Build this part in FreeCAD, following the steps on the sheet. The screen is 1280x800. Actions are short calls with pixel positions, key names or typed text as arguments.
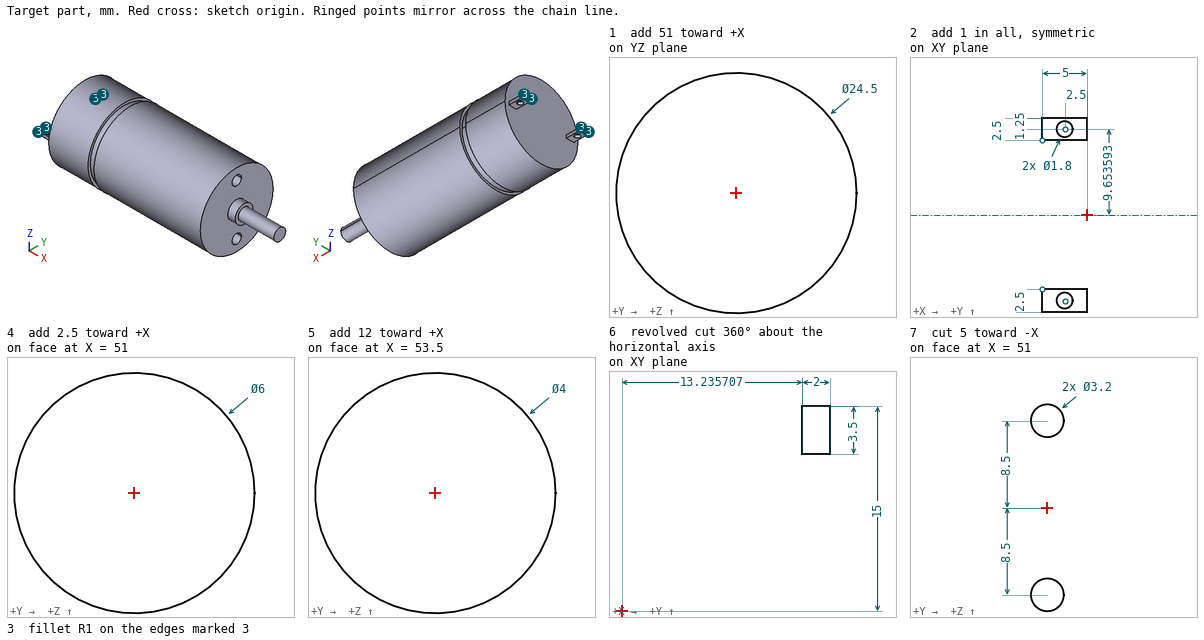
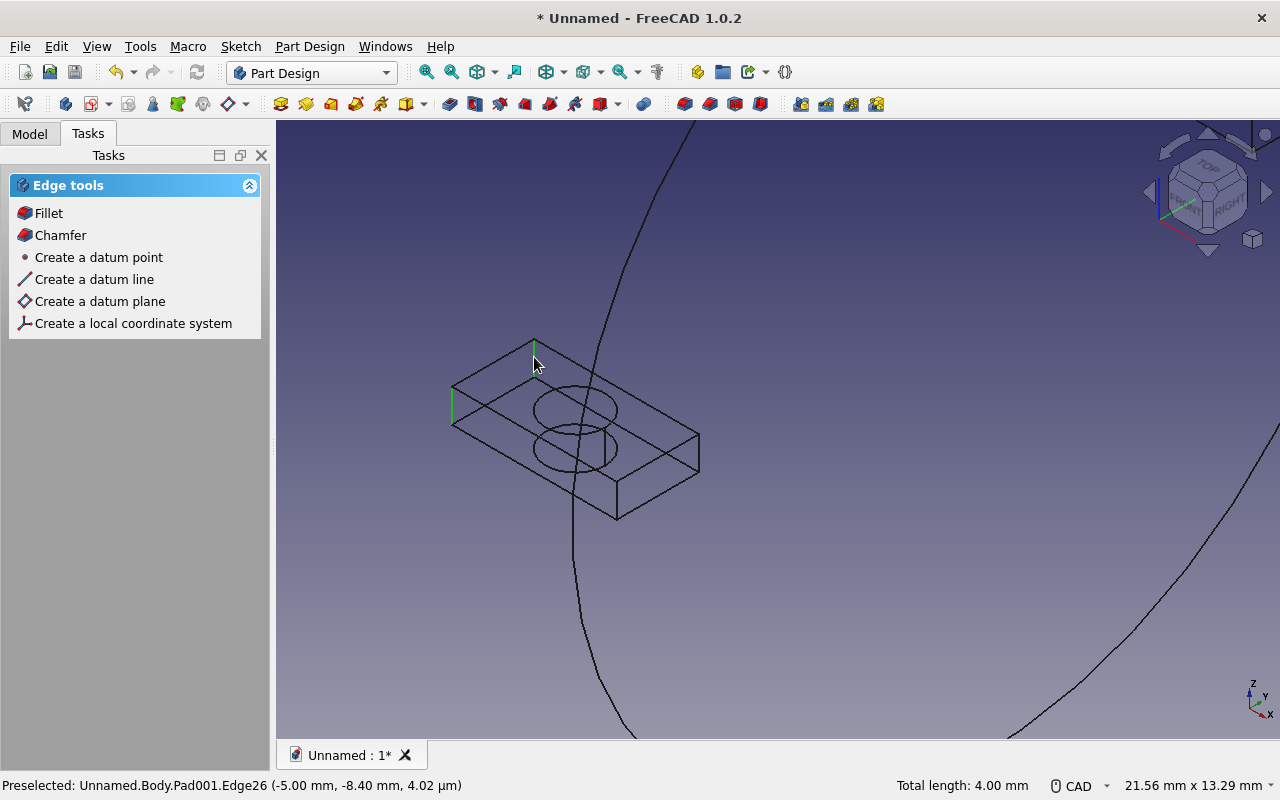
key(v)
key(1)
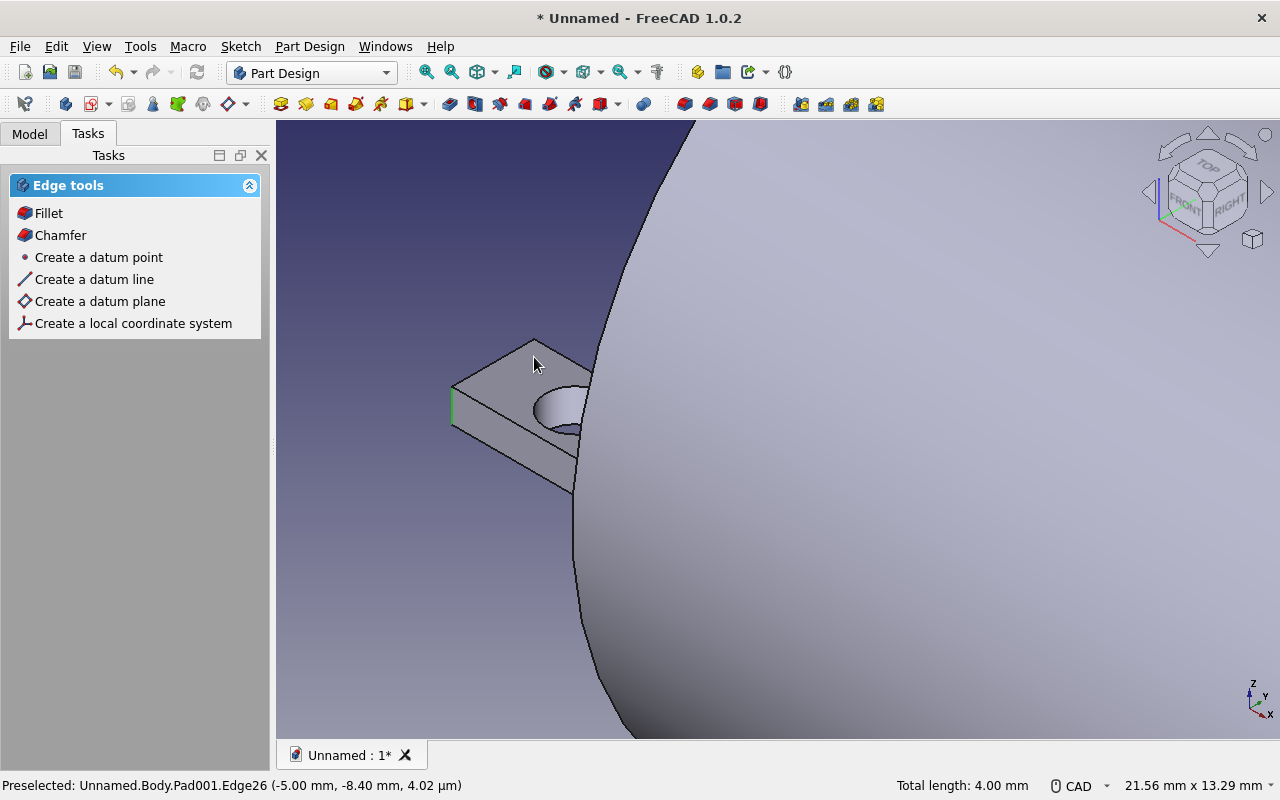
click(685, 104)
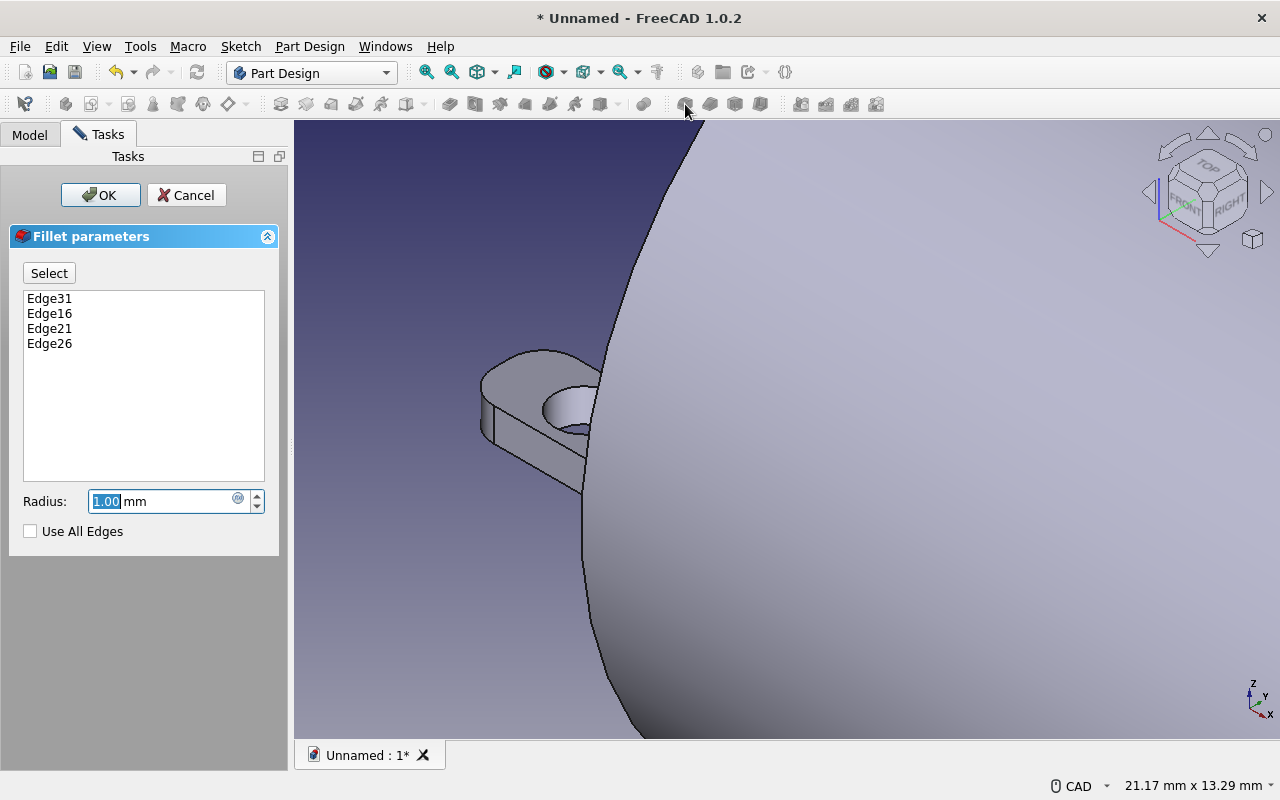
text(1)
key(Tab)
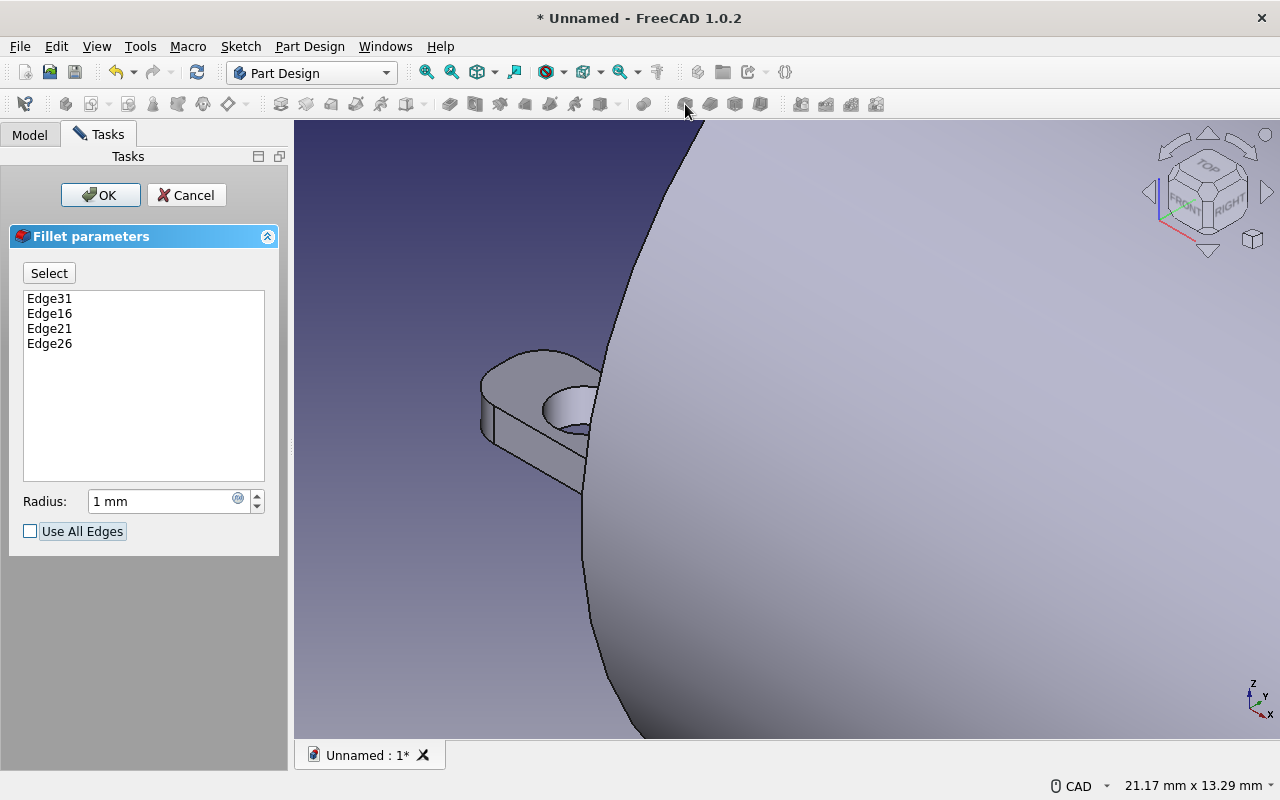
click(101, 195)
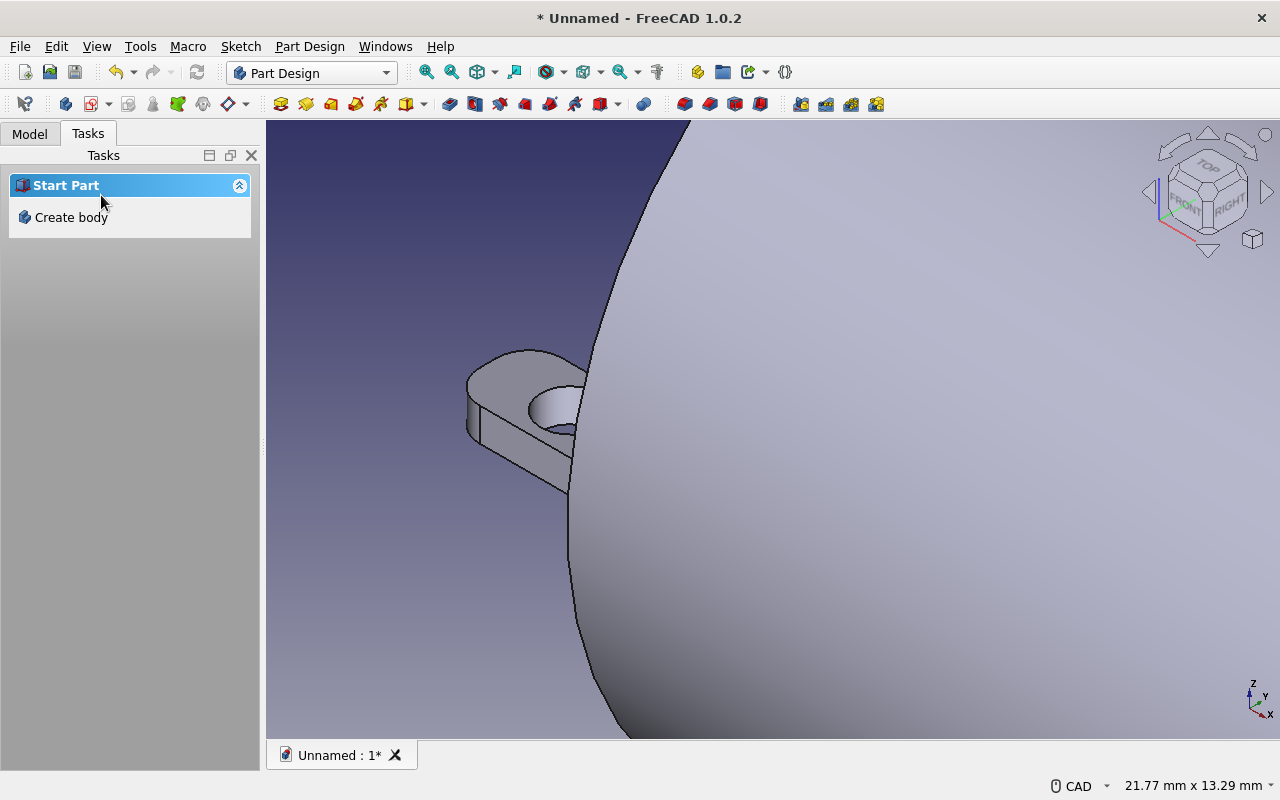
click(427, 72)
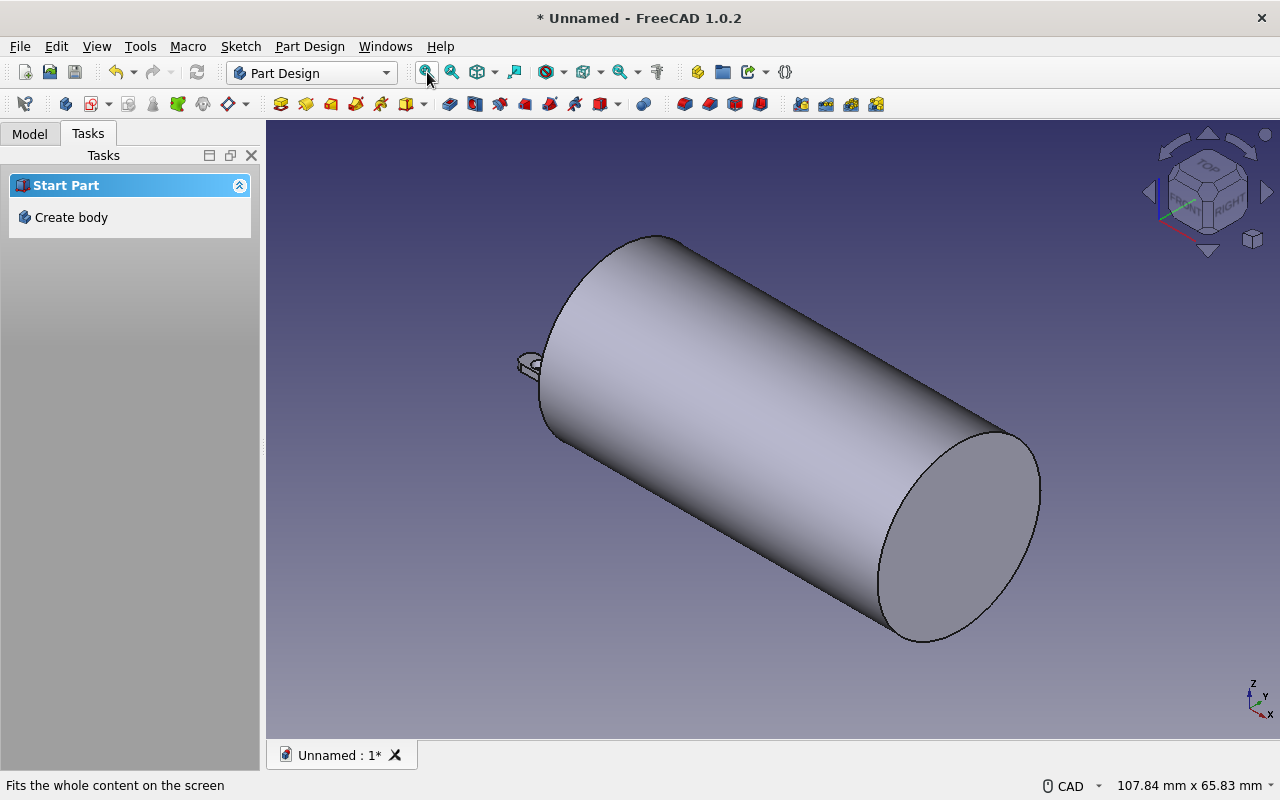
click(959, 536)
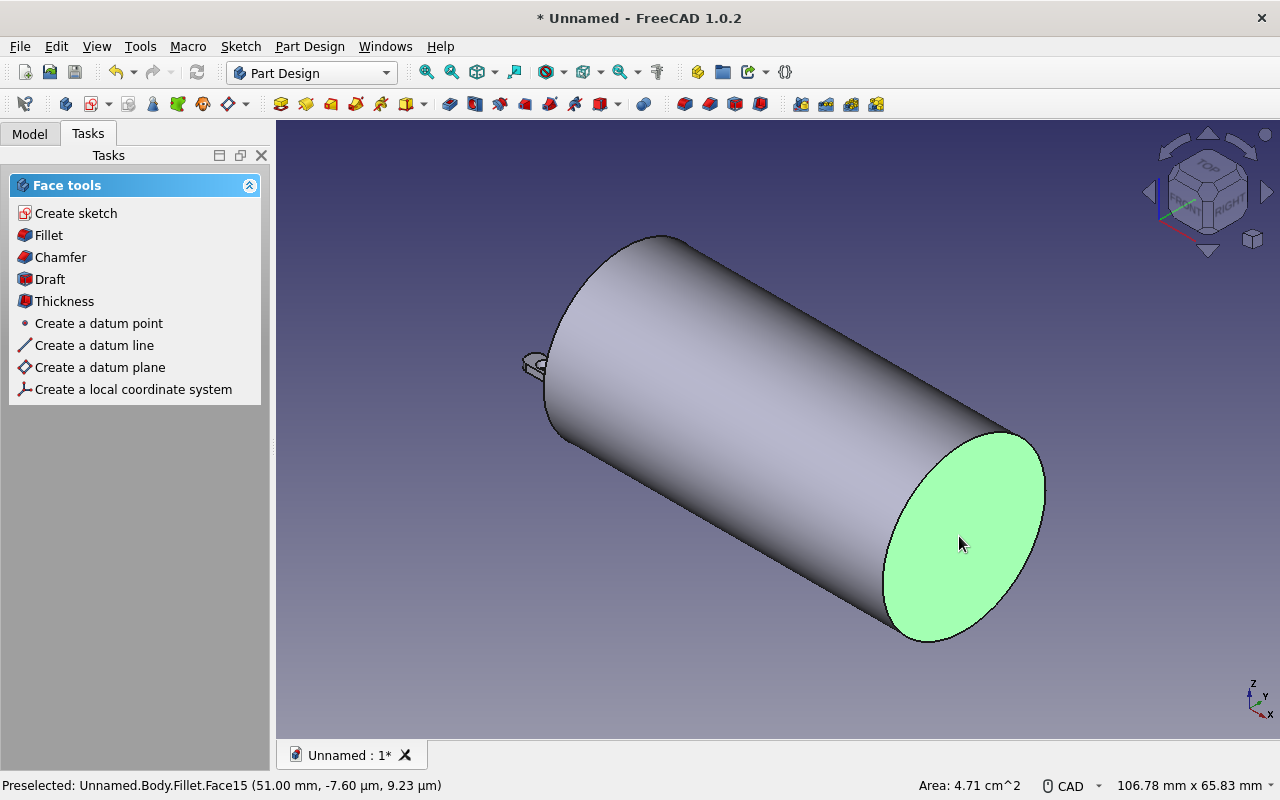
click(90, 104)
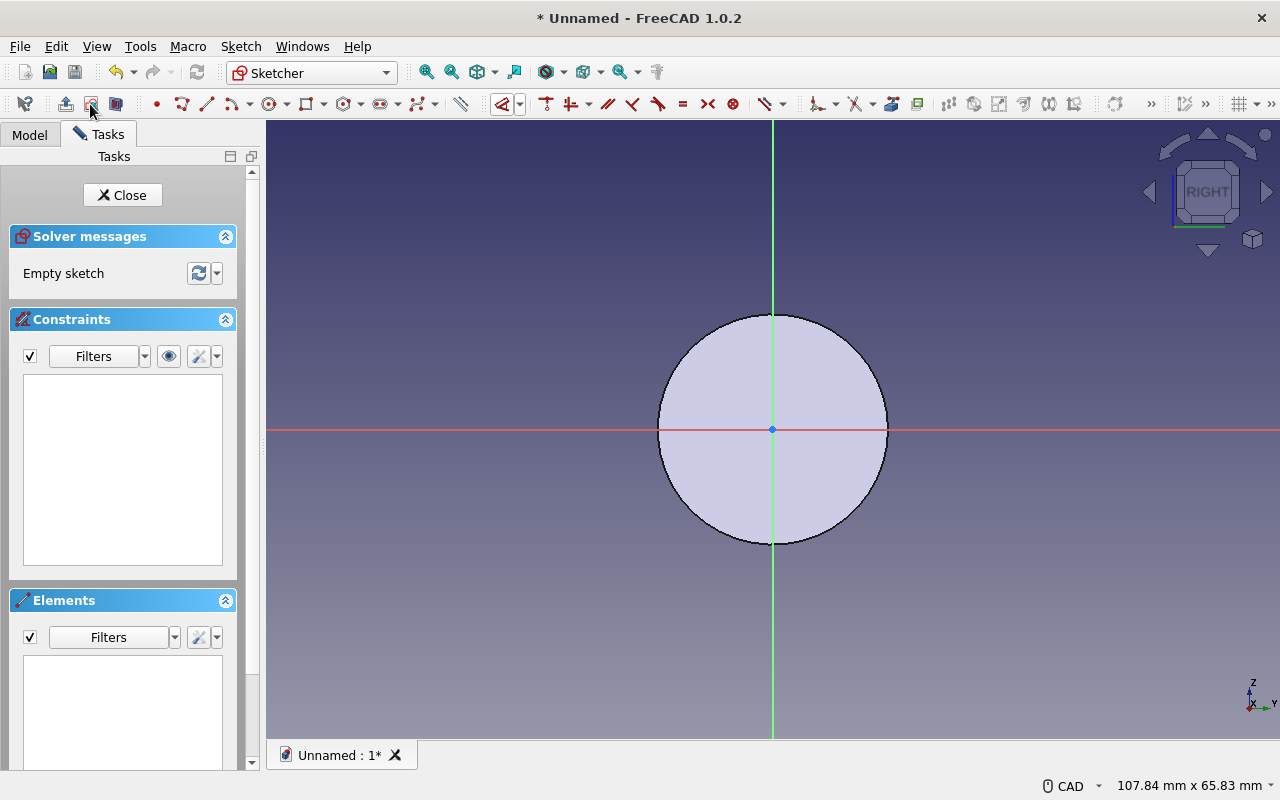
scroll(784, 429, up, 10)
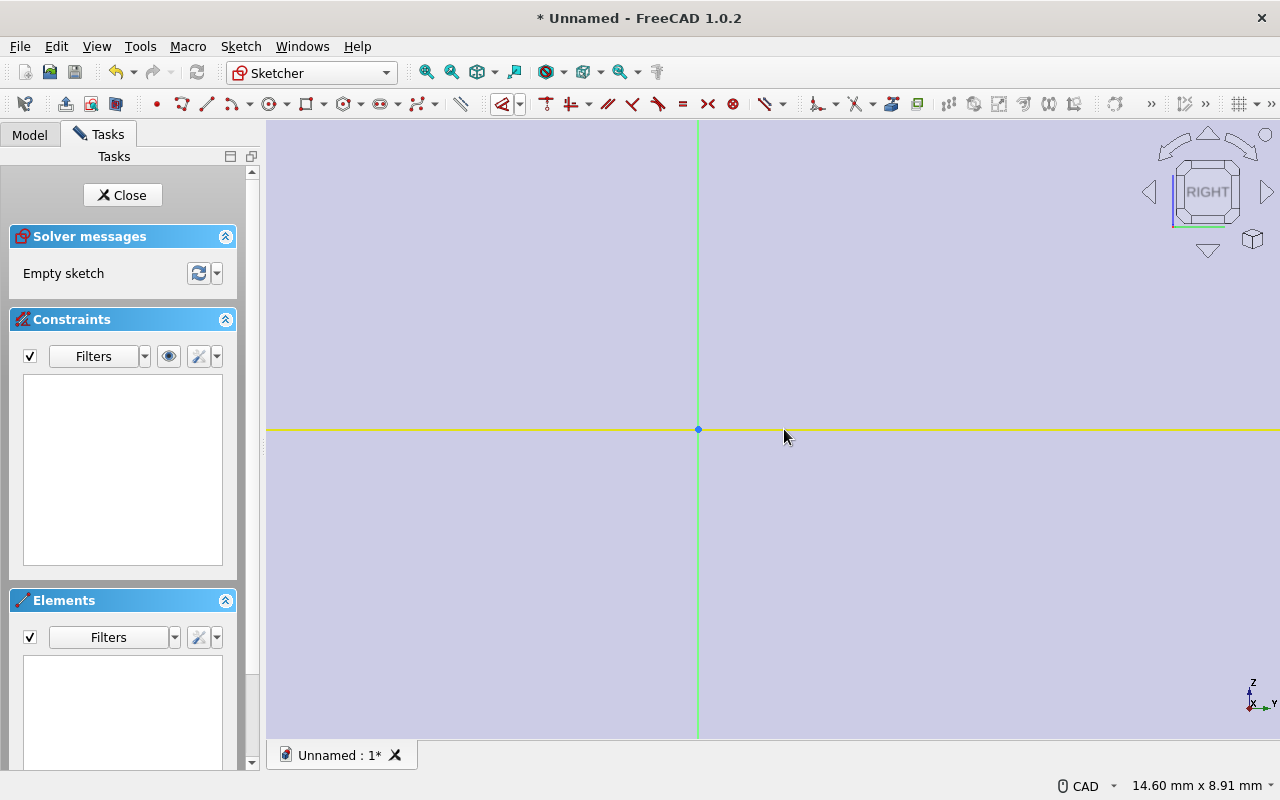
click(268, 104)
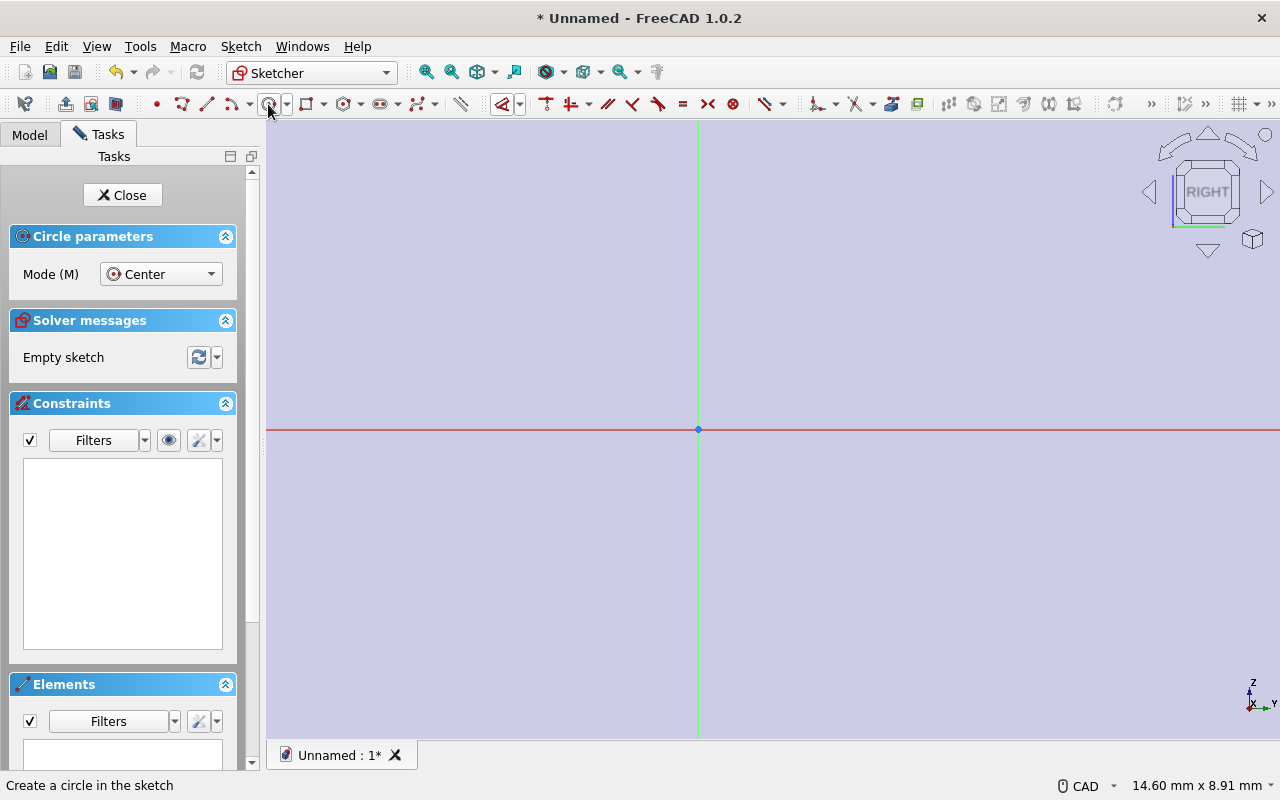
click(698, 429)
move(846, 282)